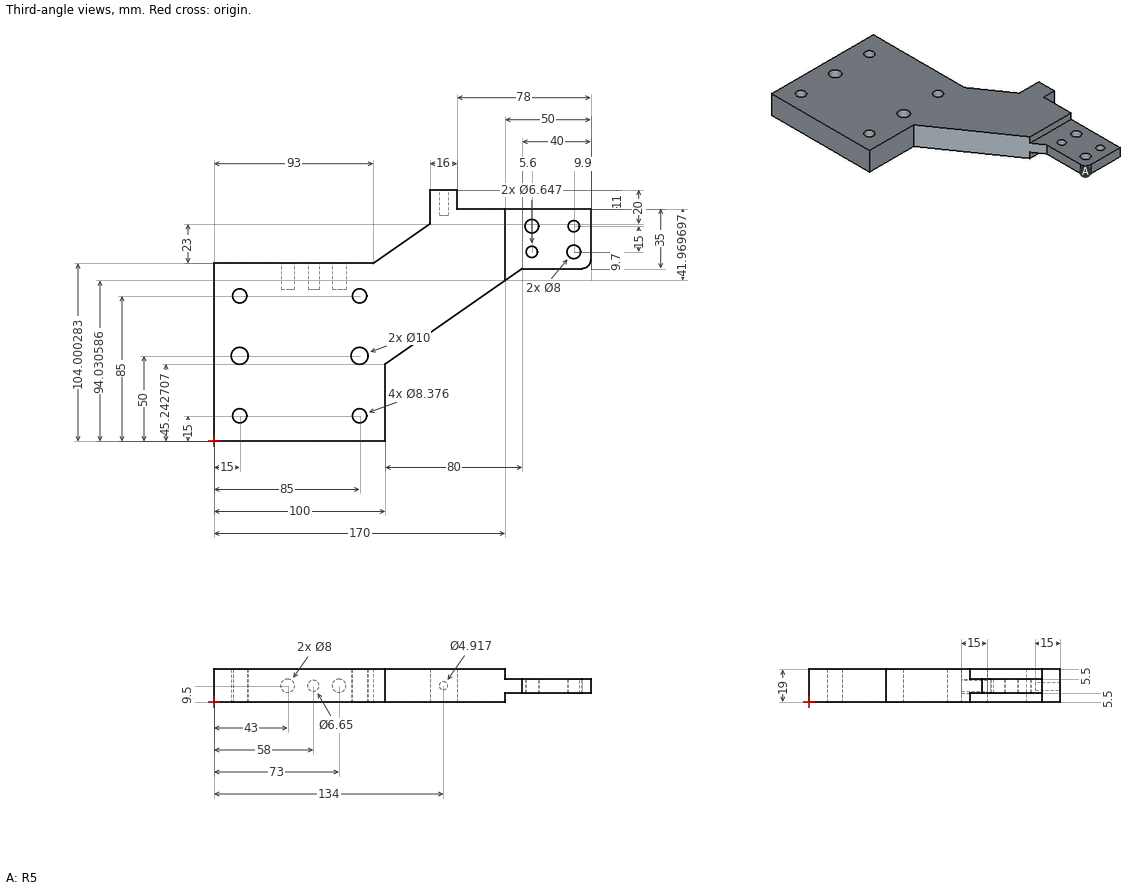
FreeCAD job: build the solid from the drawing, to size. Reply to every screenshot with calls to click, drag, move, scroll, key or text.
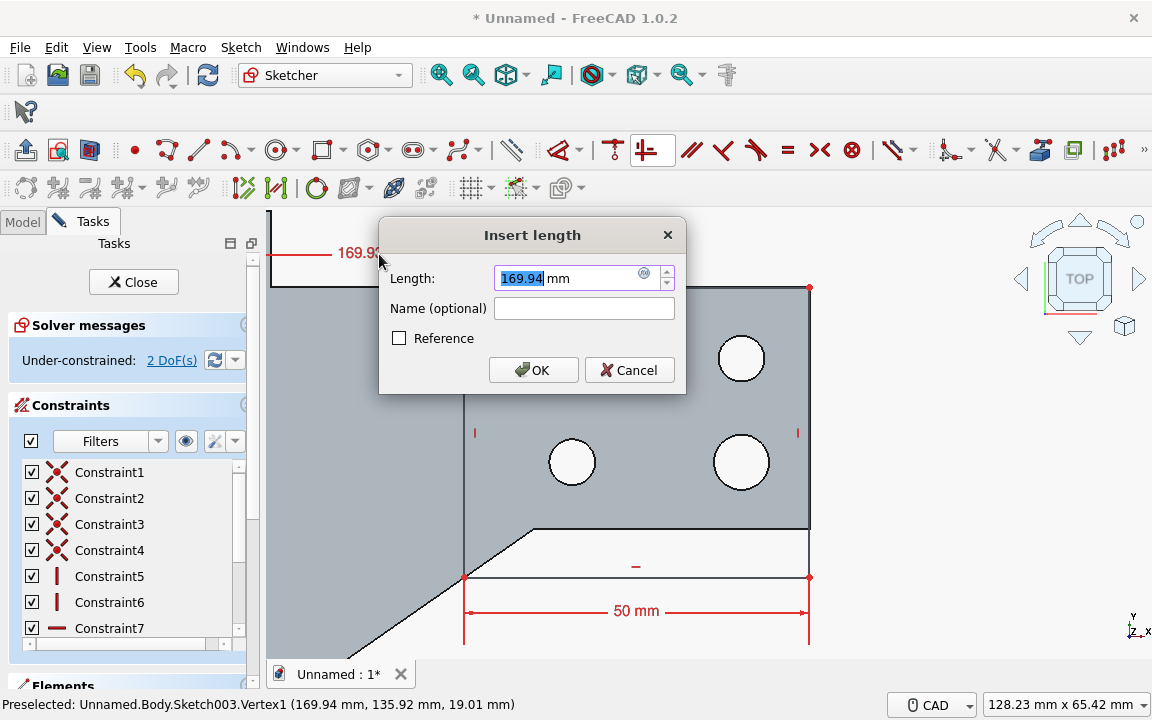
text(170)
key(Return)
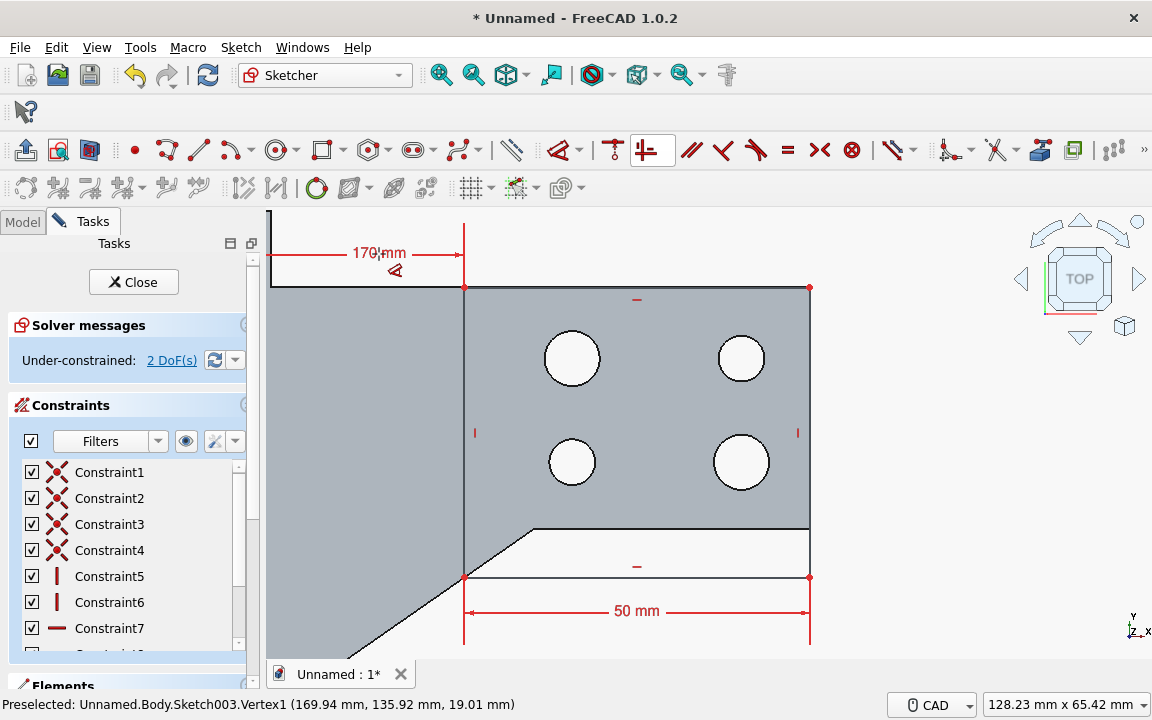
click(464, 375)
click(430, 433)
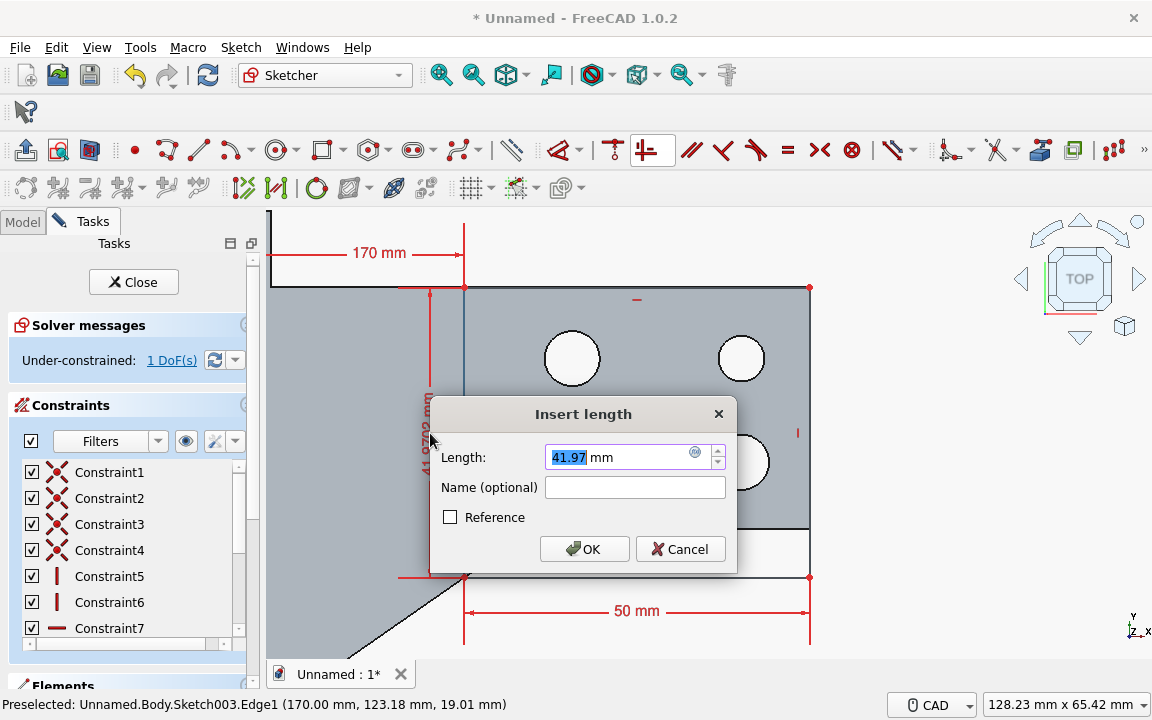
text(41.969697)
key(Return)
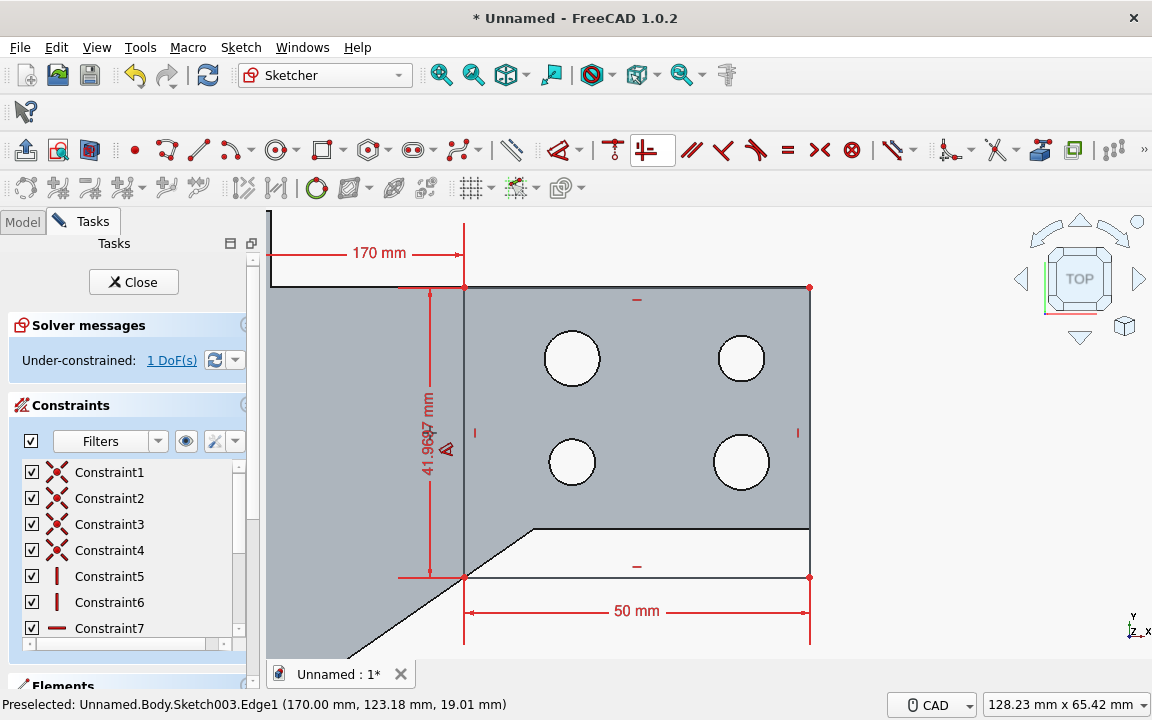
click(464, 578)
click(498, 604)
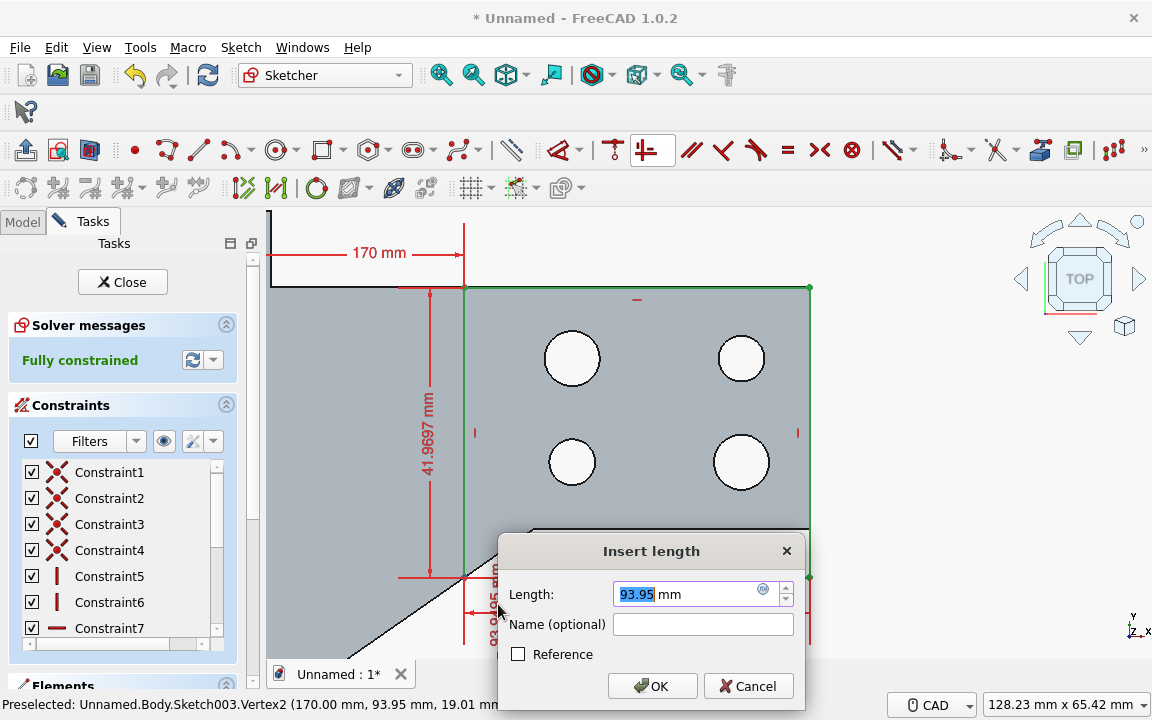
text(94.030586)
key(Return)
key(Escape)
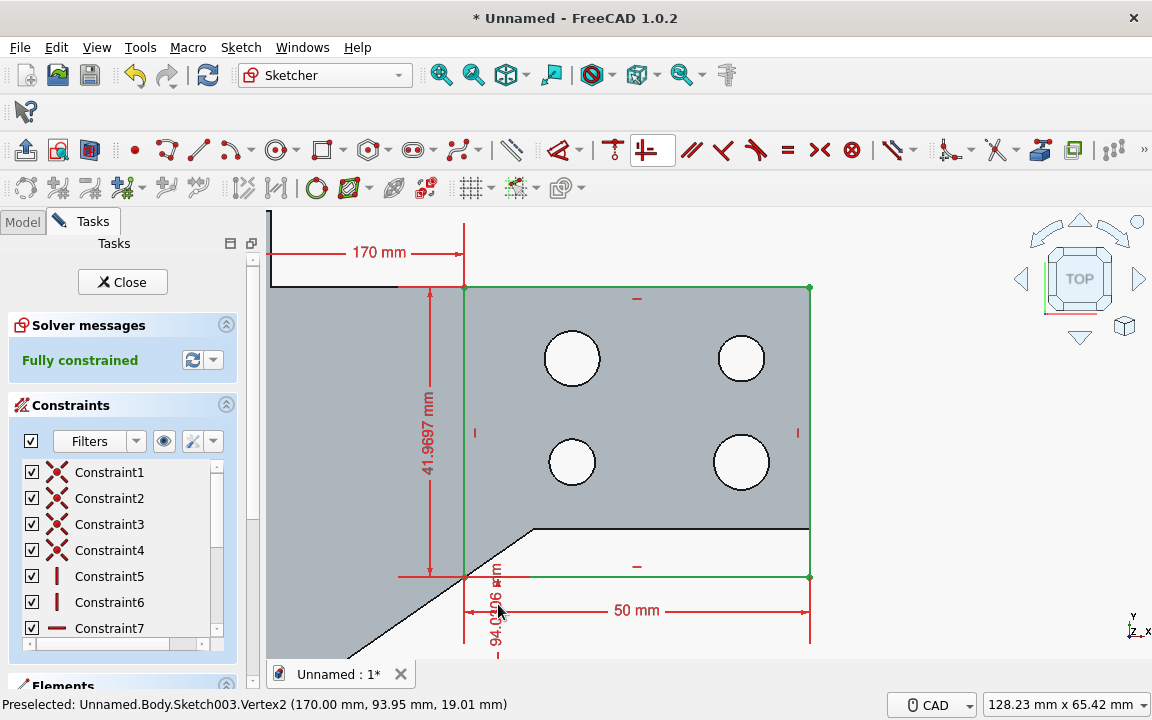
click(123, 282)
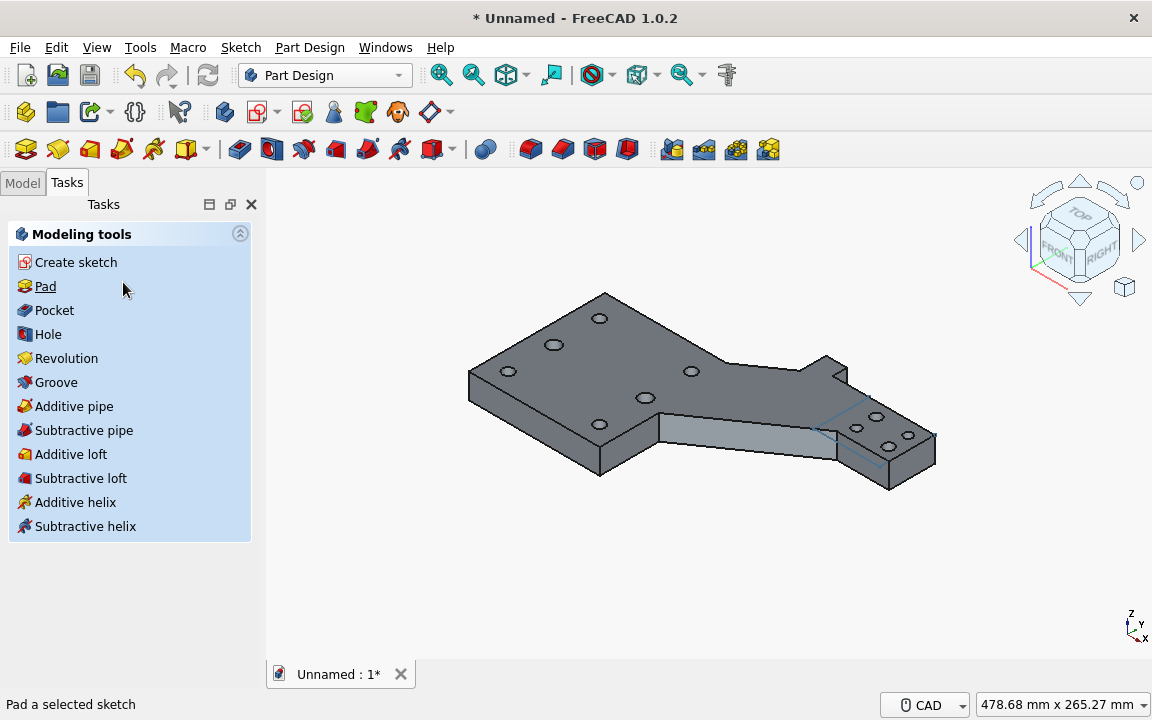
click(240, 150)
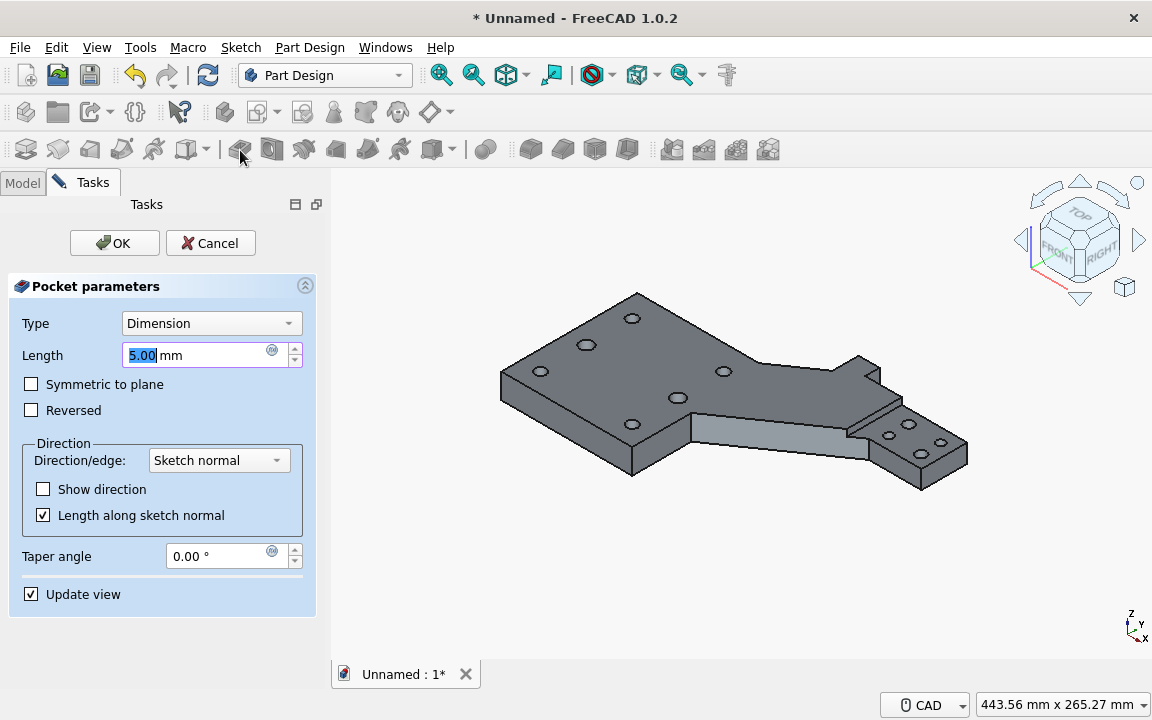
text(5.5)
key(Tab)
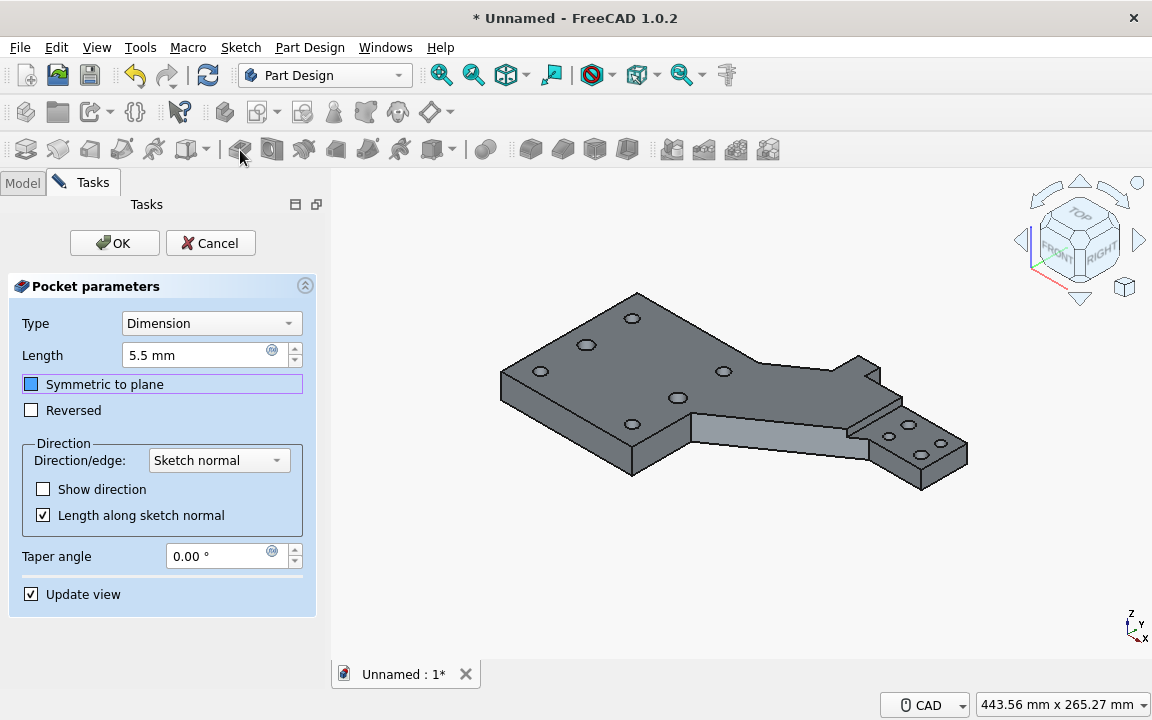
click(115, 243)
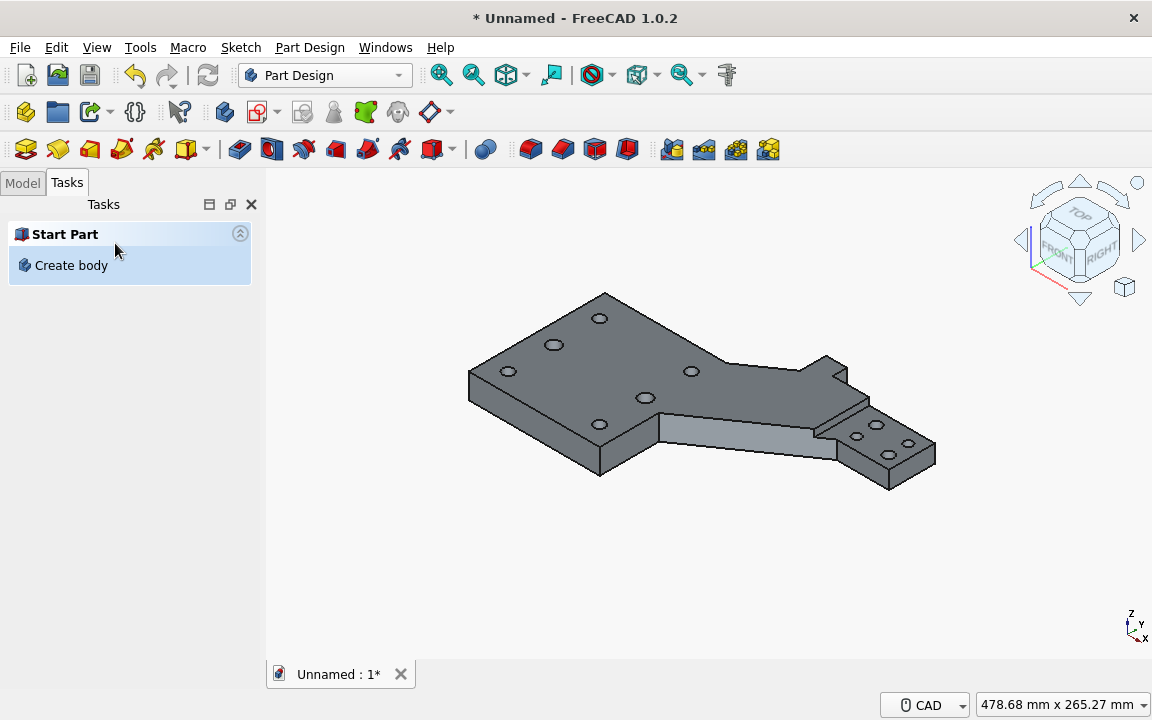
click(258, 112)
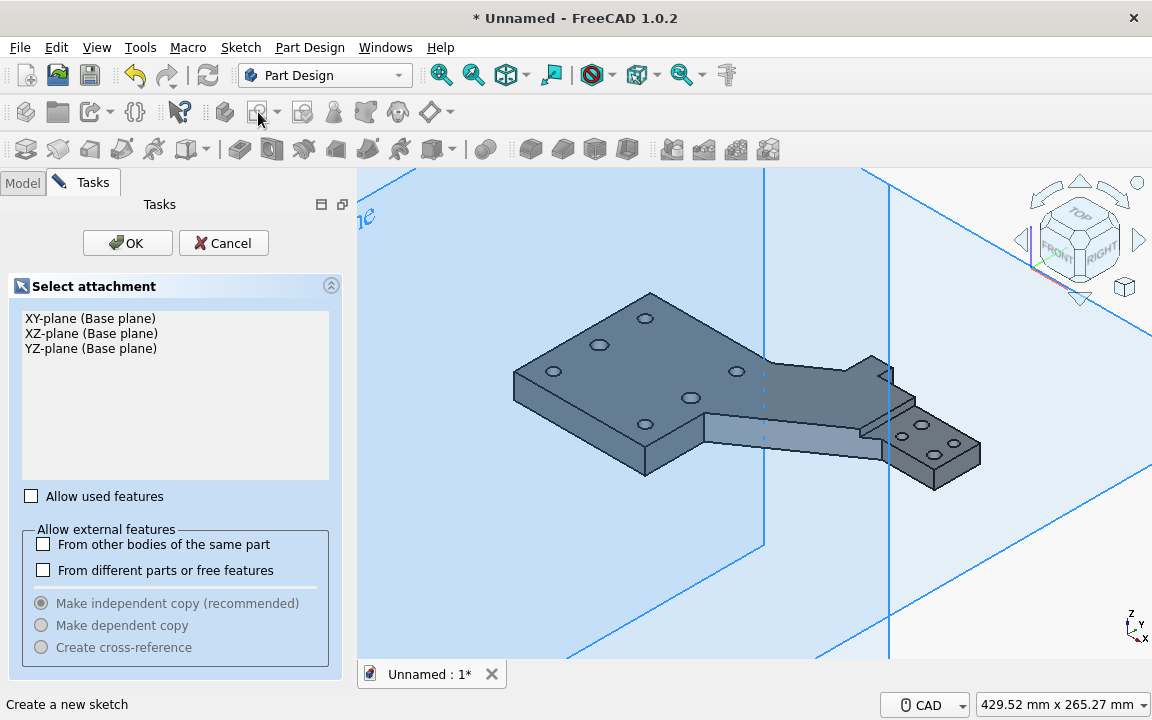
click(82, 318)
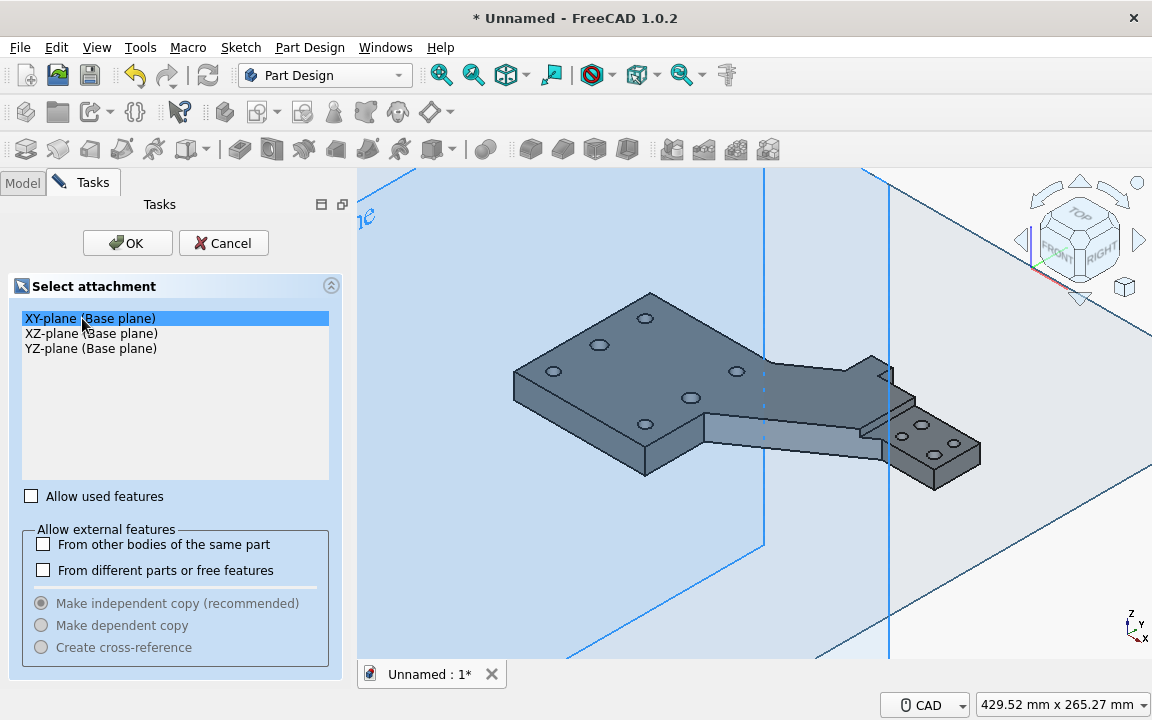
click(128, 243)